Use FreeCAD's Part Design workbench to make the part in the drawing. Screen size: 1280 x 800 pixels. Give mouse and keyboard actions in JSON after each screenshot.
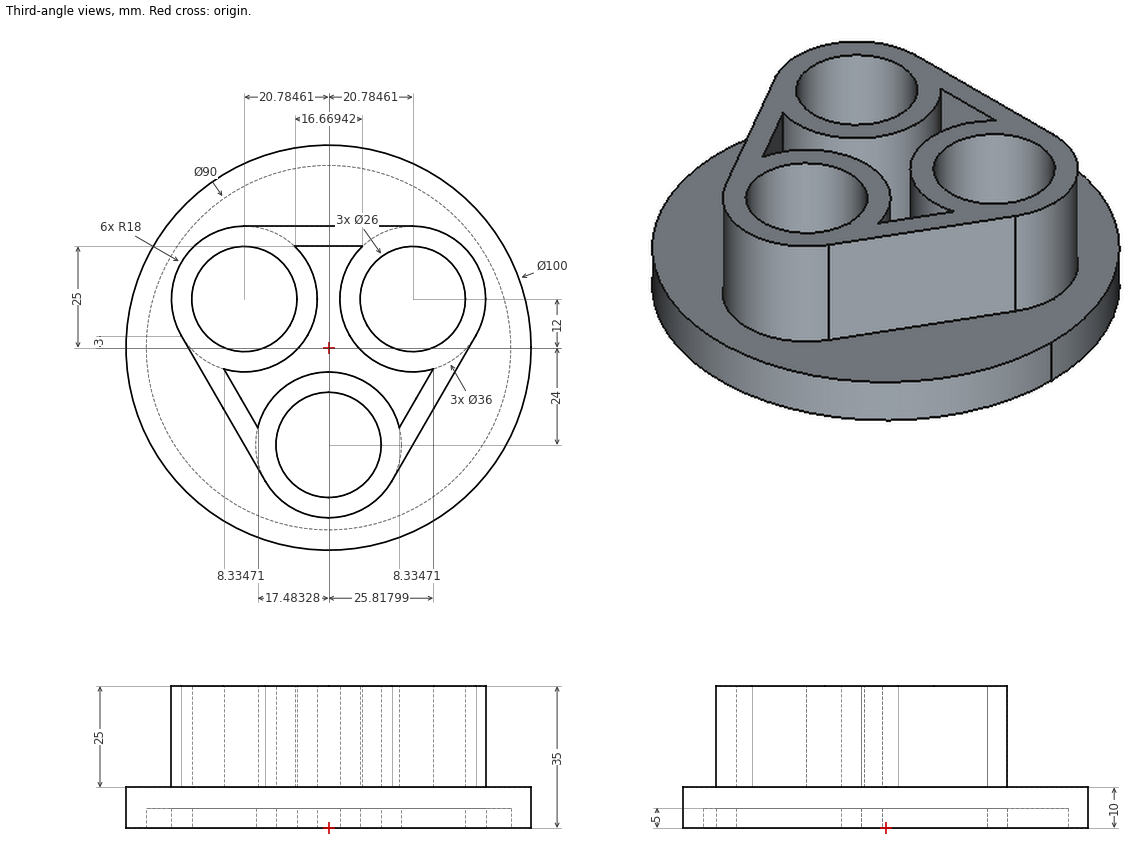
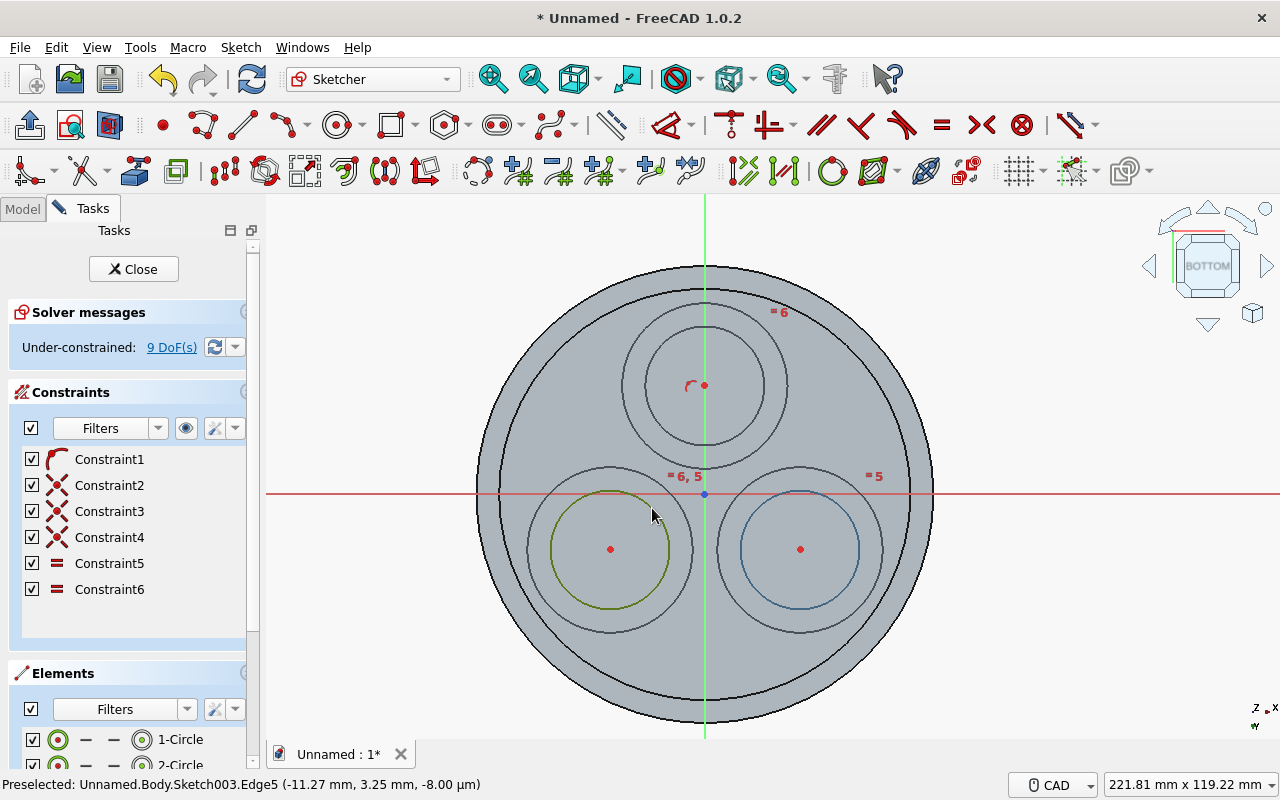
{"action": "left_click", "coordinate": [747, 344]}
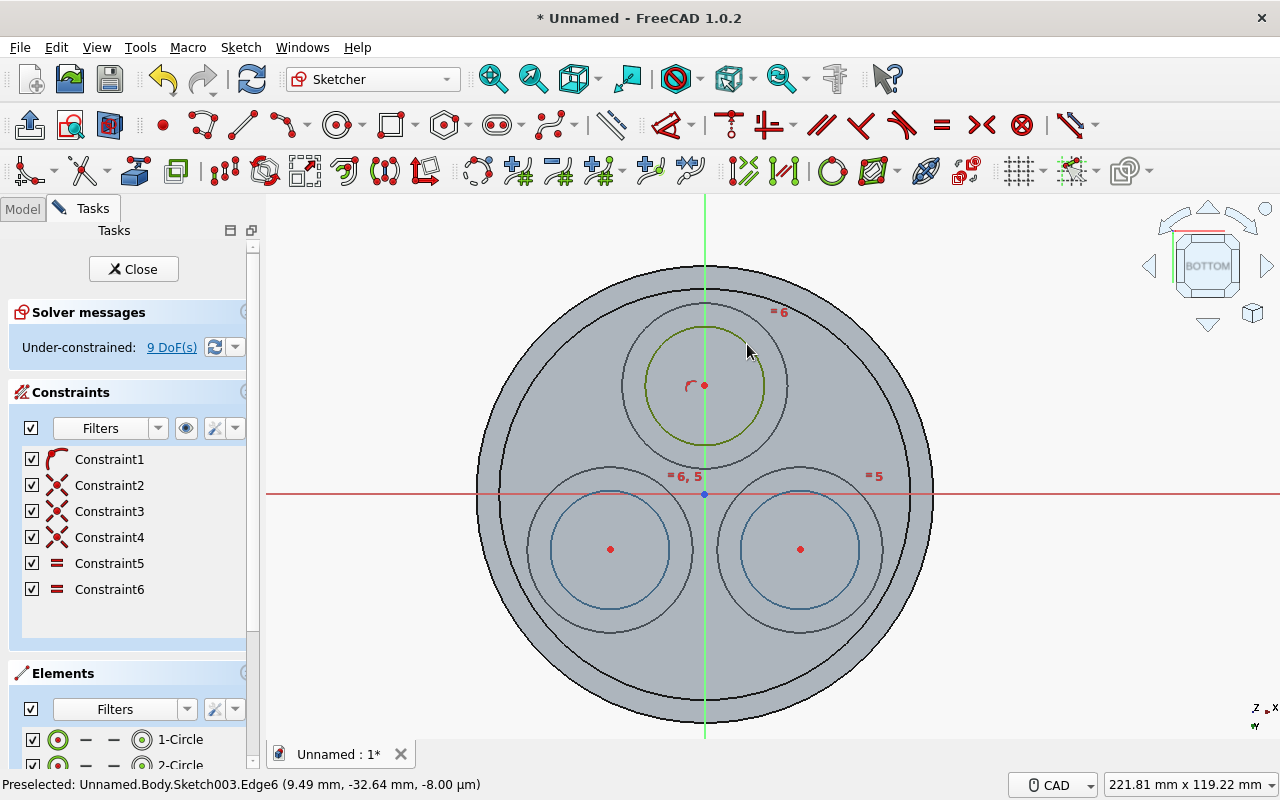
{"action": "key", "text": "e"}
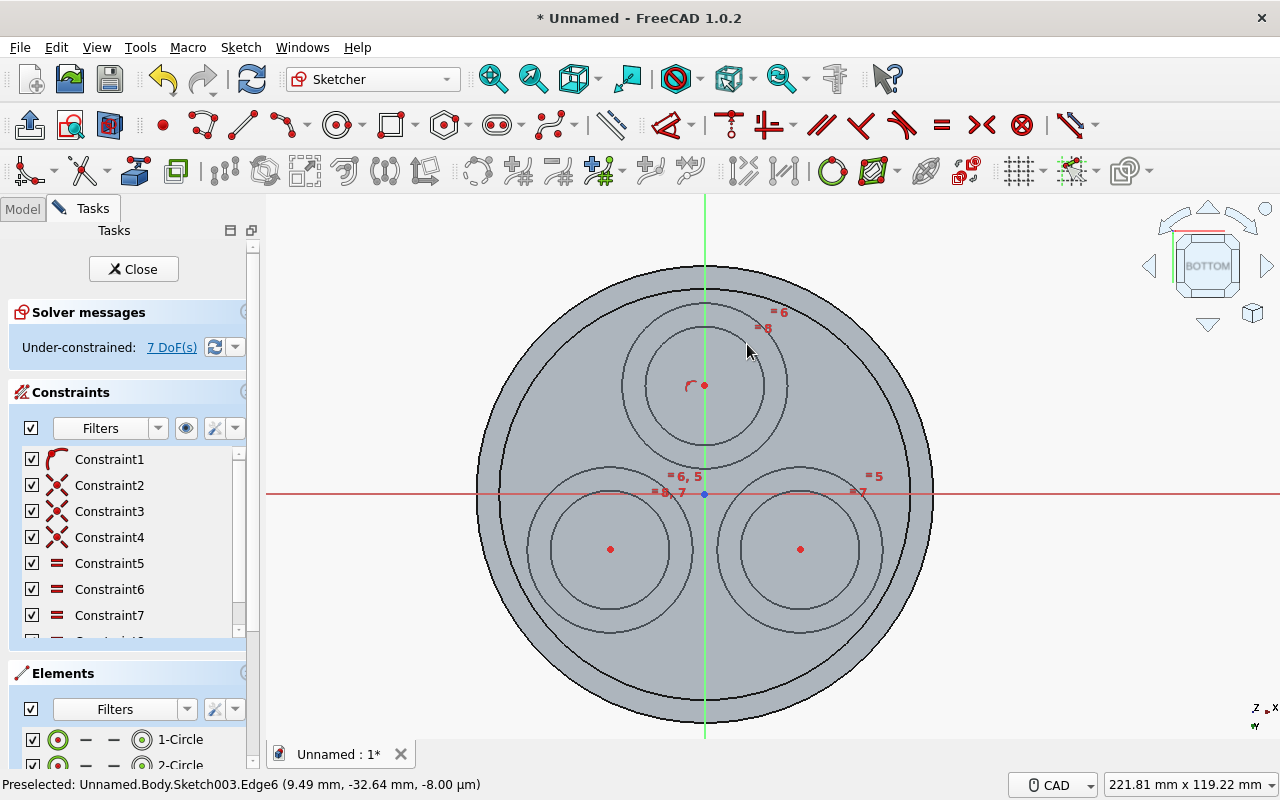
{"action": "left_click", "coordinate": [800, 550]}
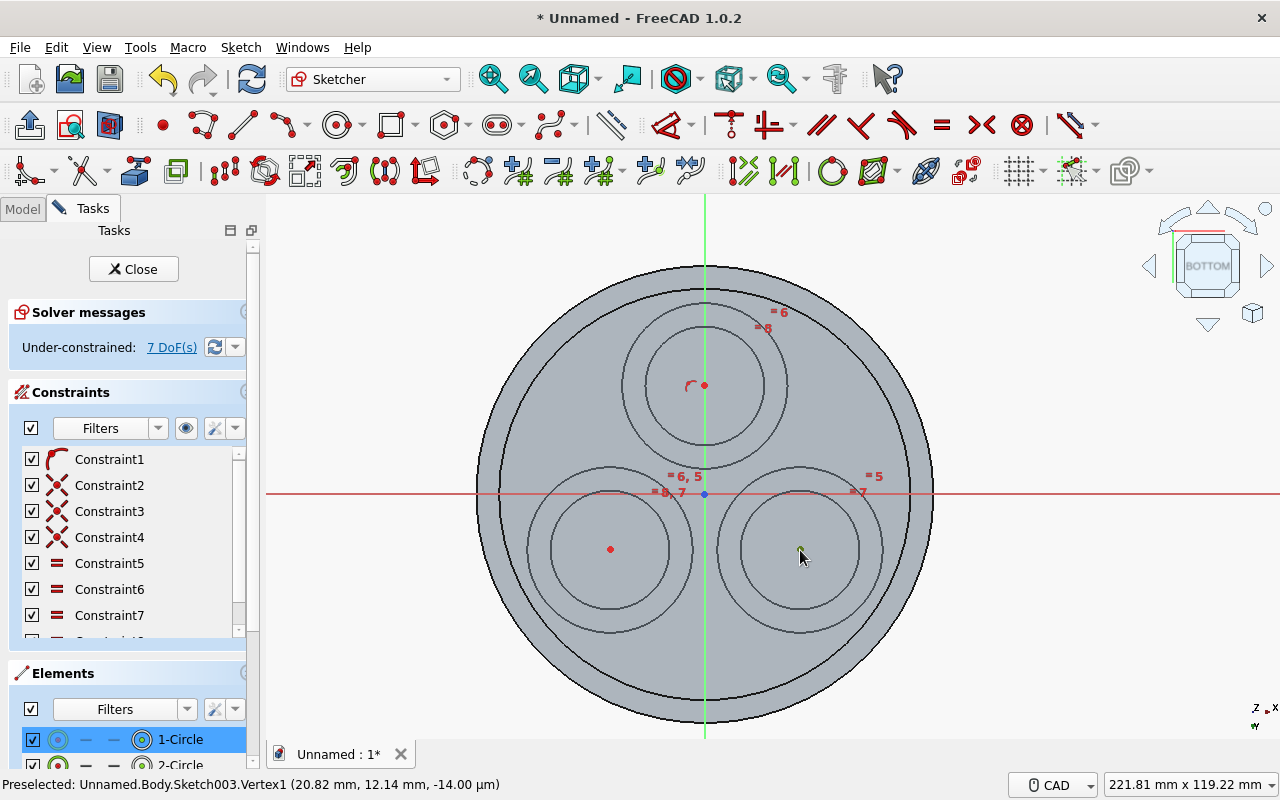
{"action": "left_click", "coordinate": [610, 550]}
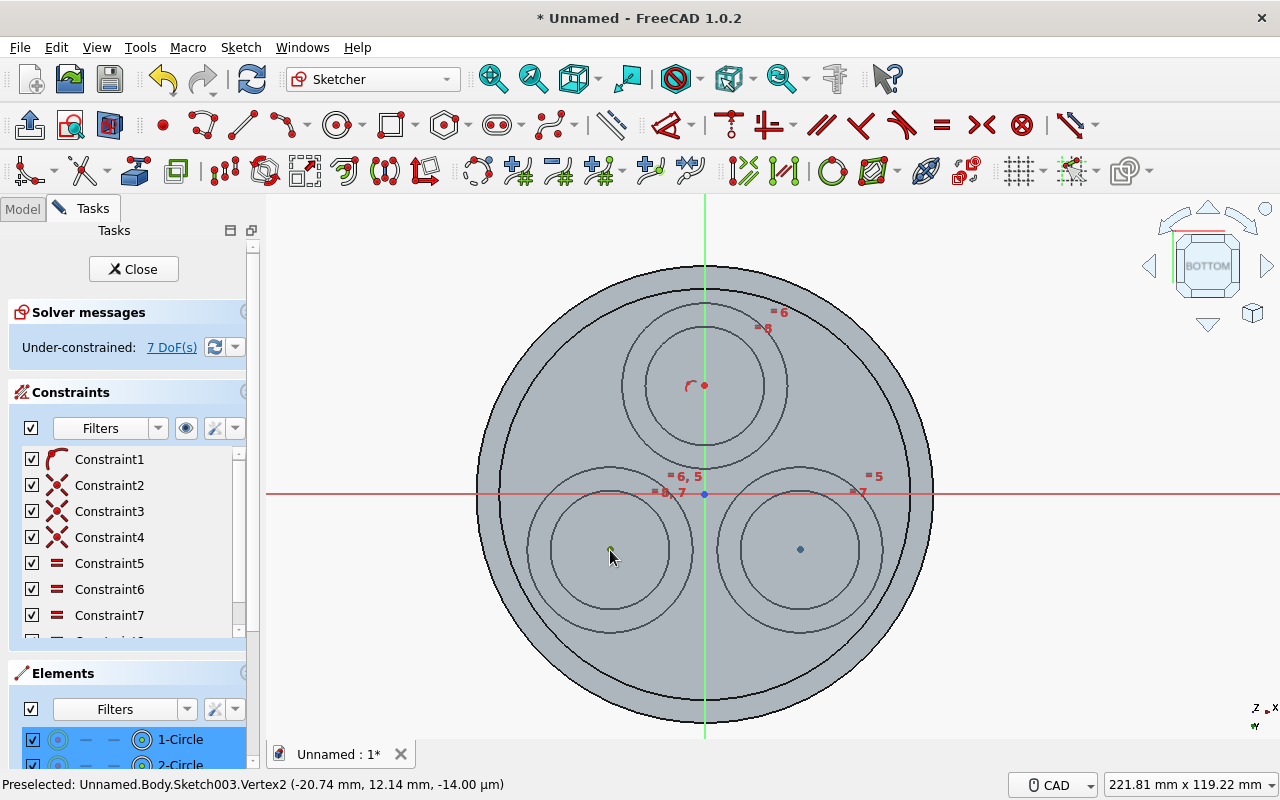
{"action": "key", "text": "h"}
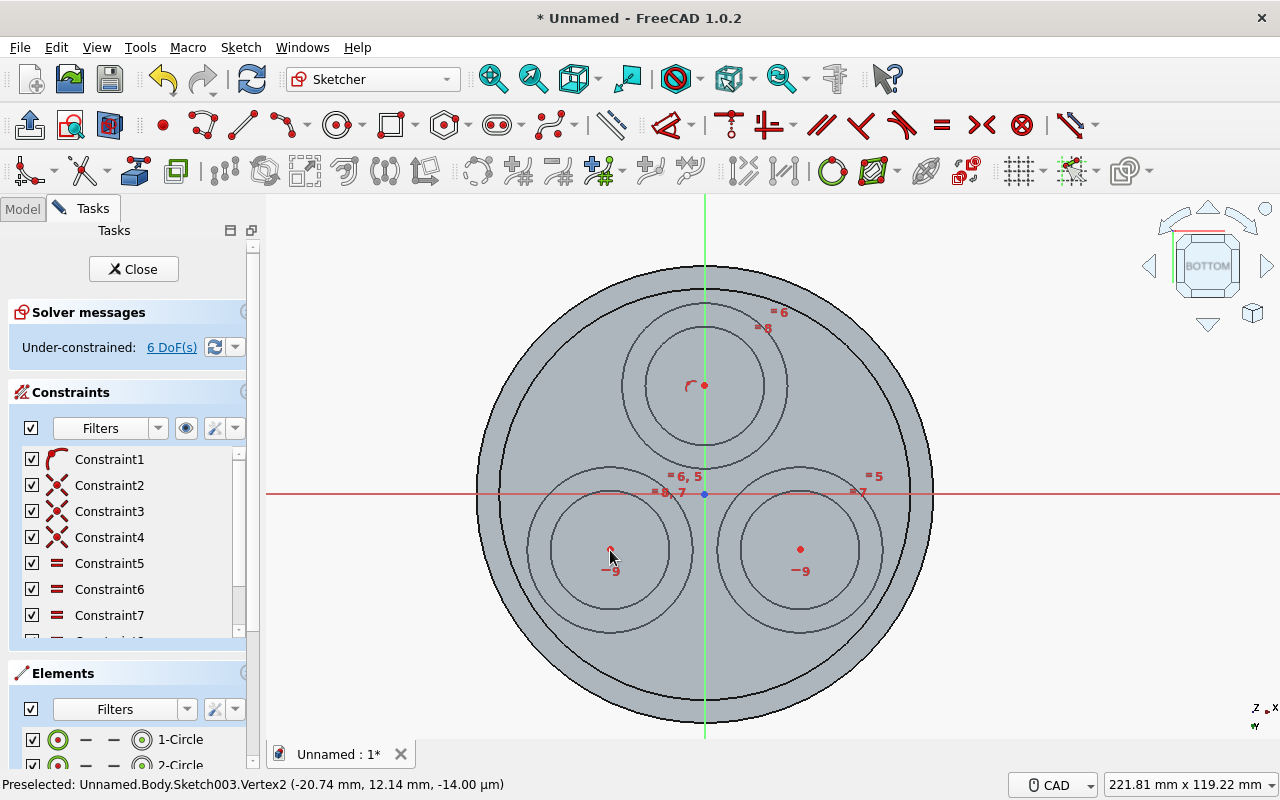
{"action": "key", "text": "d"}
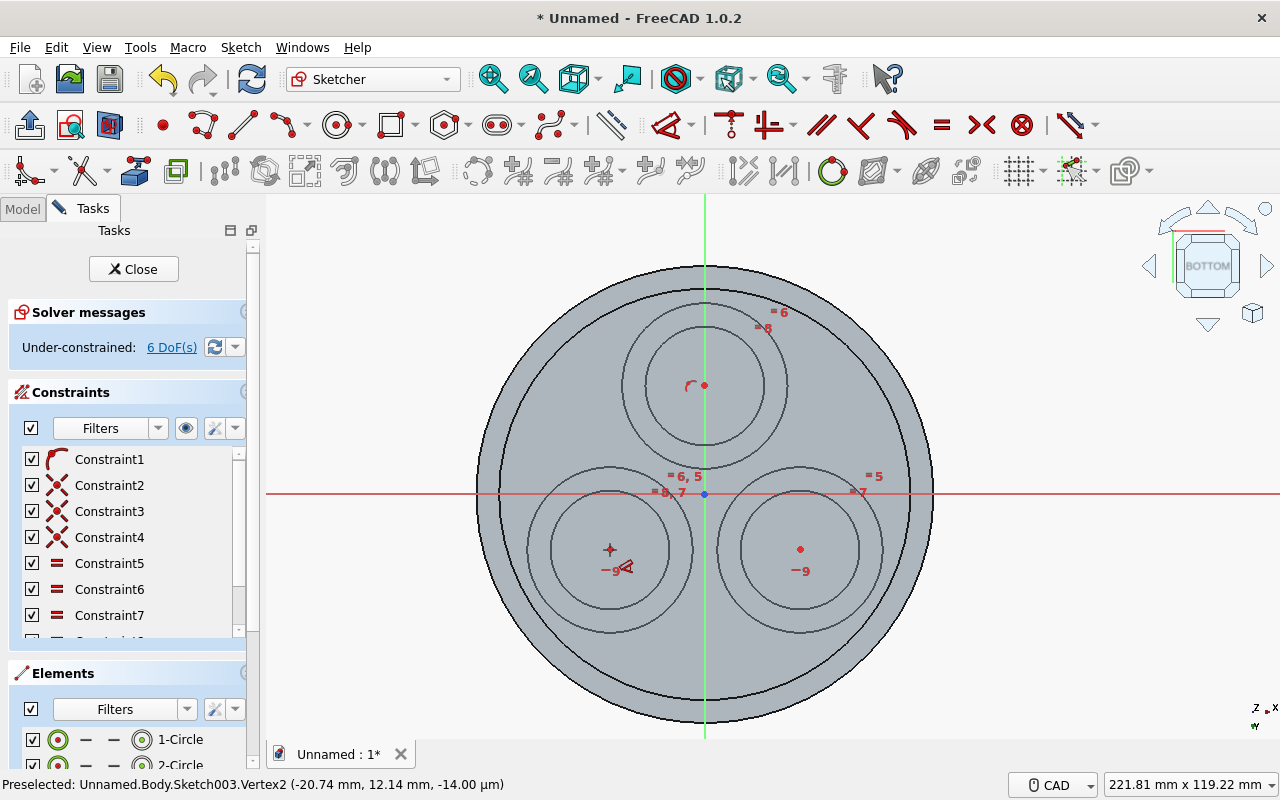
{"action": "left_click", "coordinate": [858, 491]}
{"action": "left_click", "coordinate": [880, 468]}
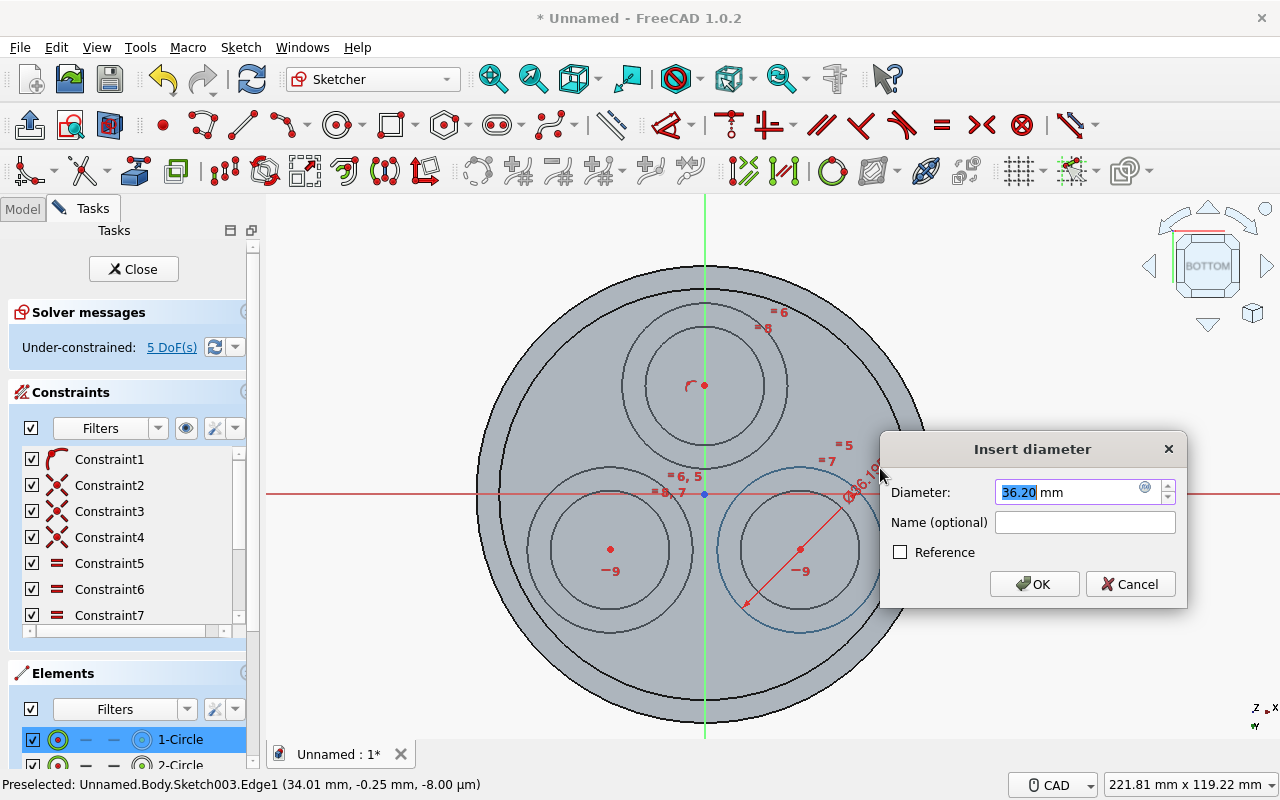
{"action": "type", "text": "36"}
{"action": "key", "text": "Return"}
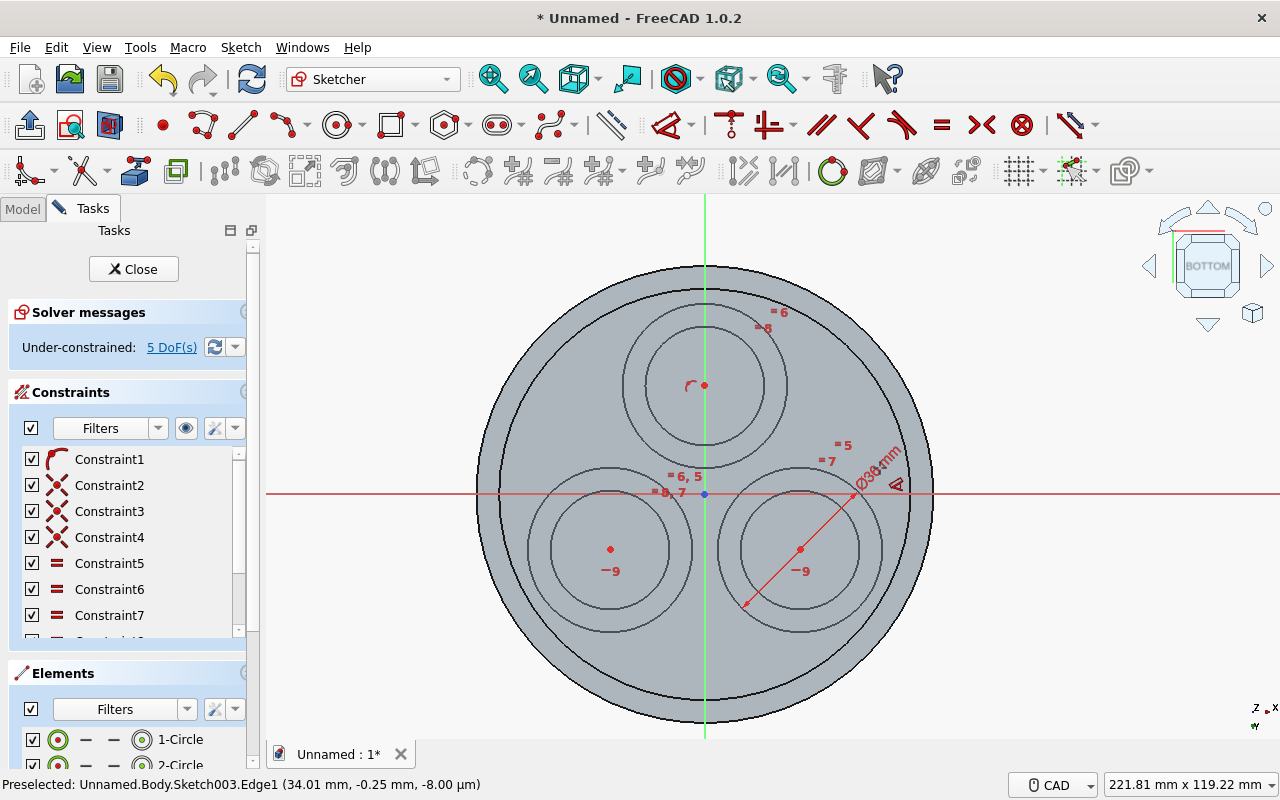
{"action": "left_click", "coordinate": [842, 508]}
{"action": "left_click", "coordinate": [910, 518]}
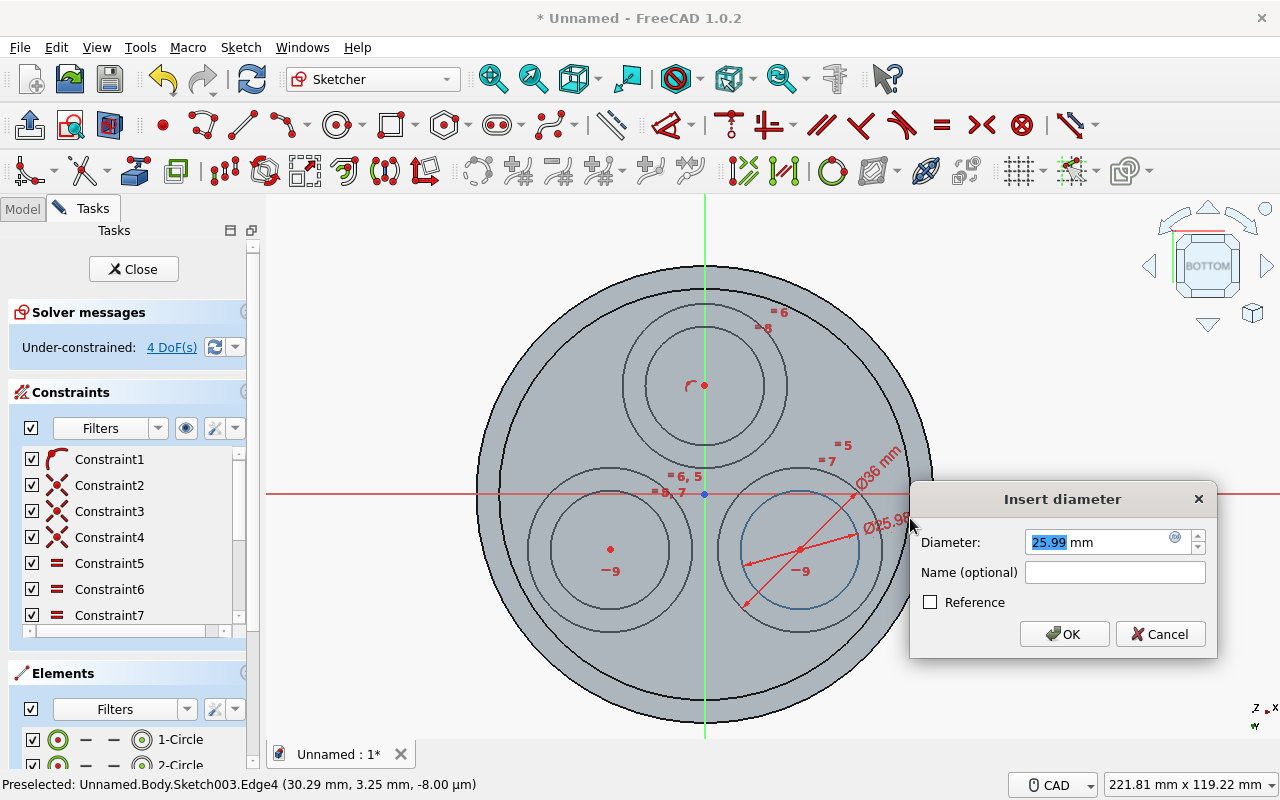
{"action": "type", "text": "26"}
{"action": "key", "text": "Return"}